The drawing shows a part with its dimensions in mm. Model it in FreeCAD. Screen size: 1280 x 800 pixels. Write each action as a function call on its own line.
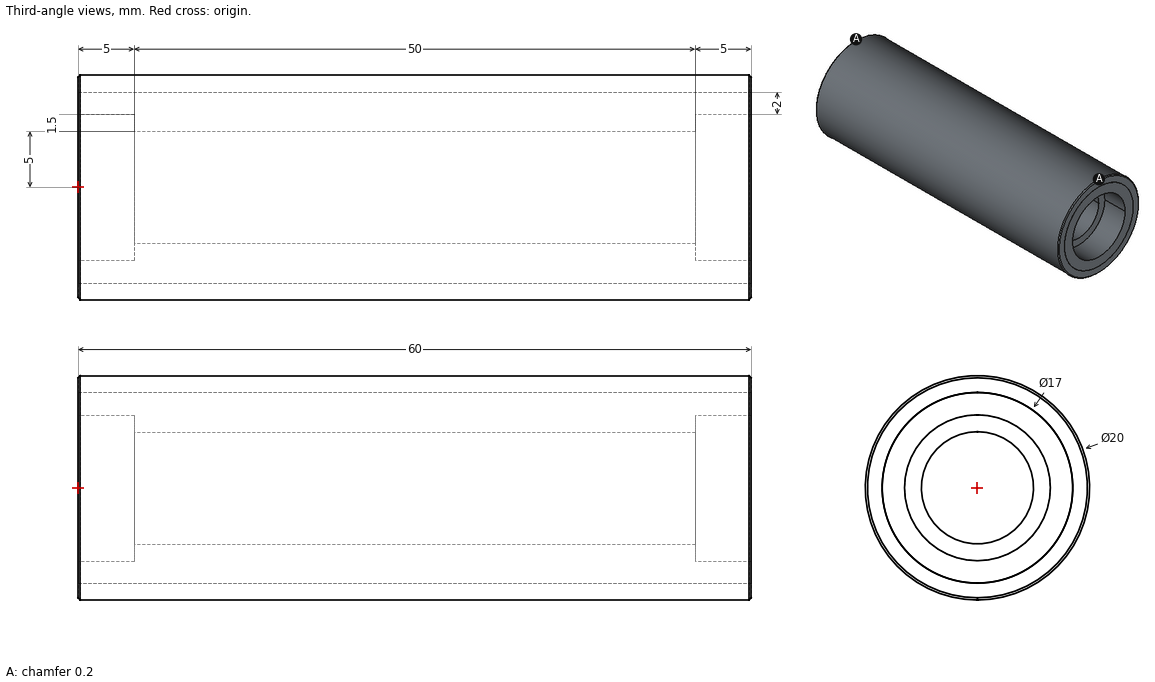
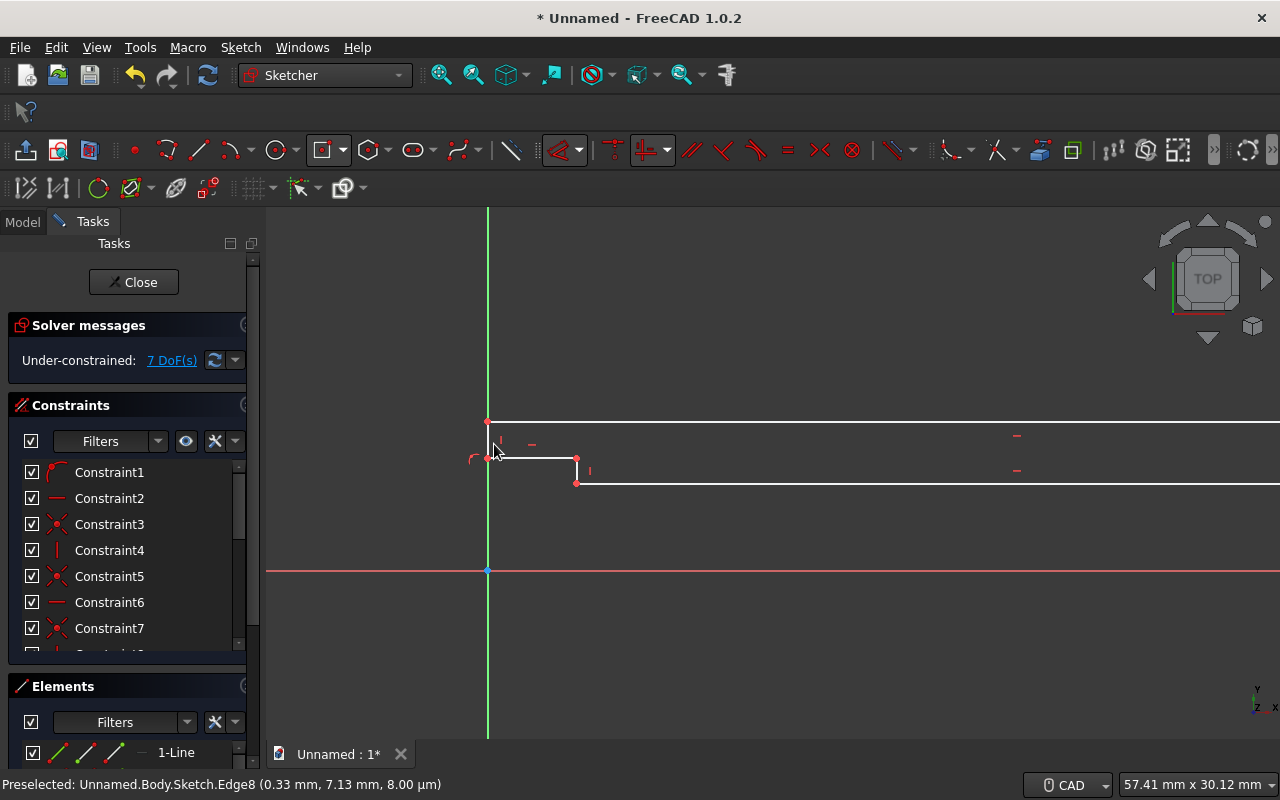
click(514, 458)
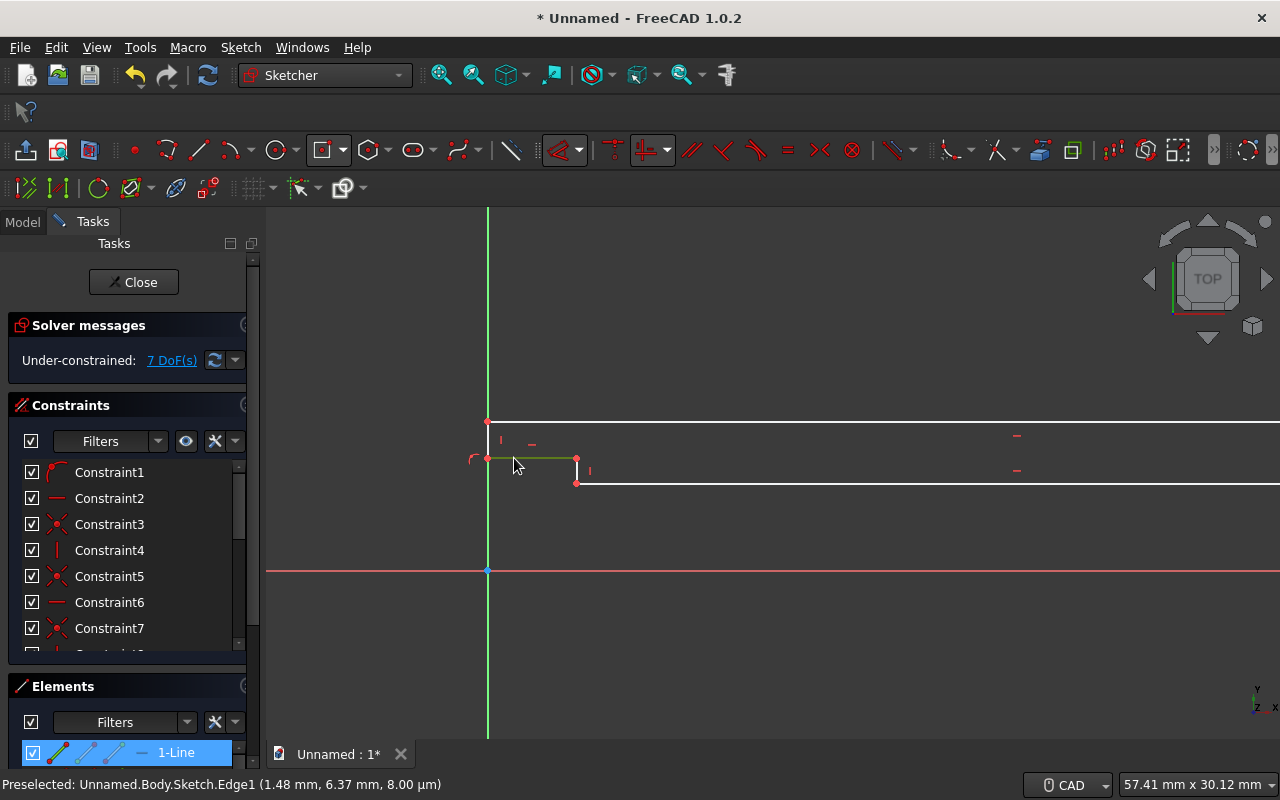
key(l)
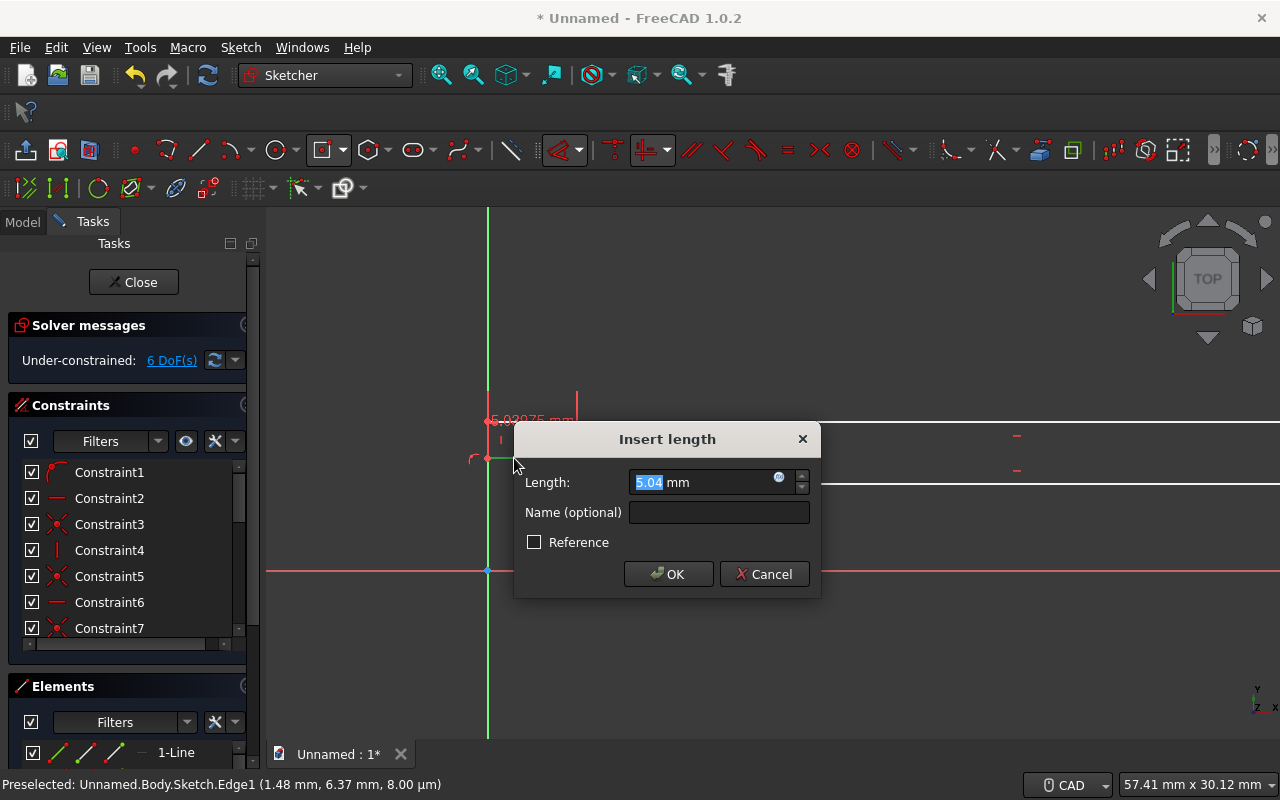
text(5)
key(Return)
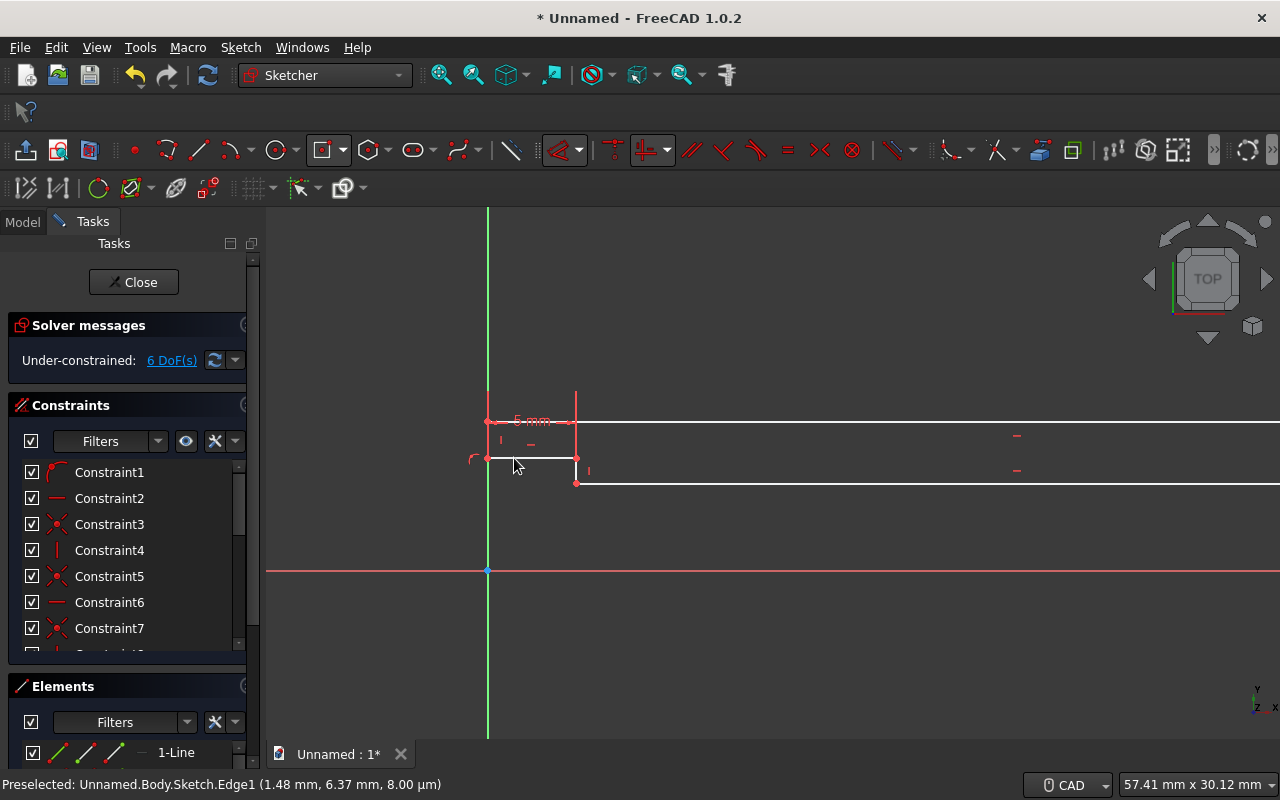
scroll(324, 445, down, 3)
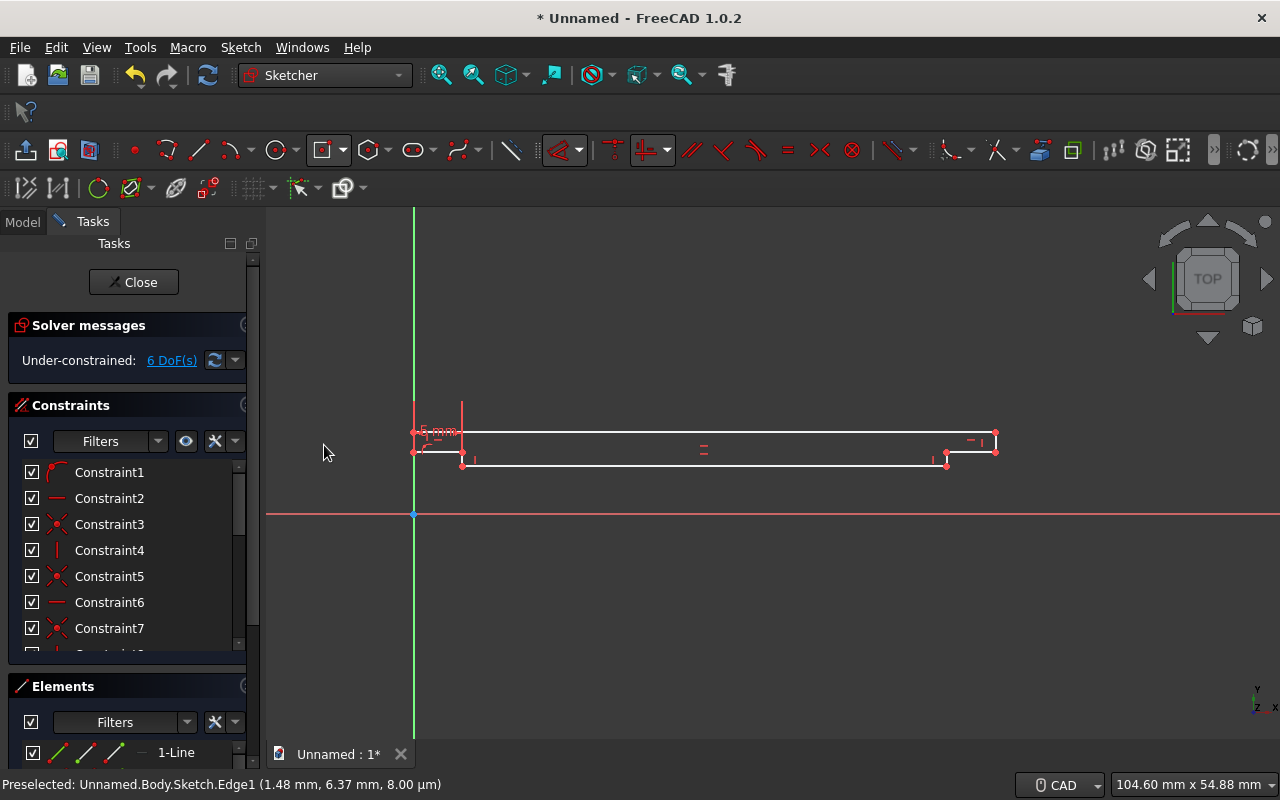
click(961, 452)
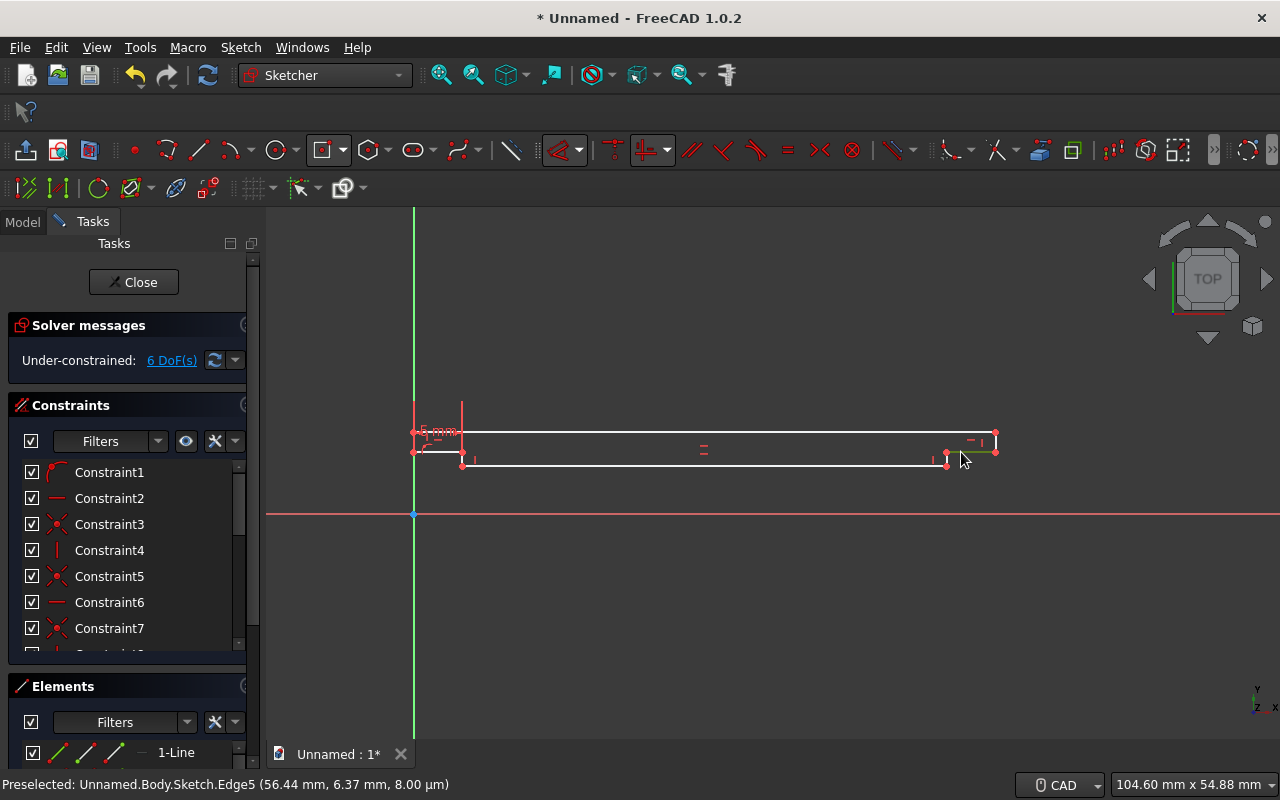
click(582, 150)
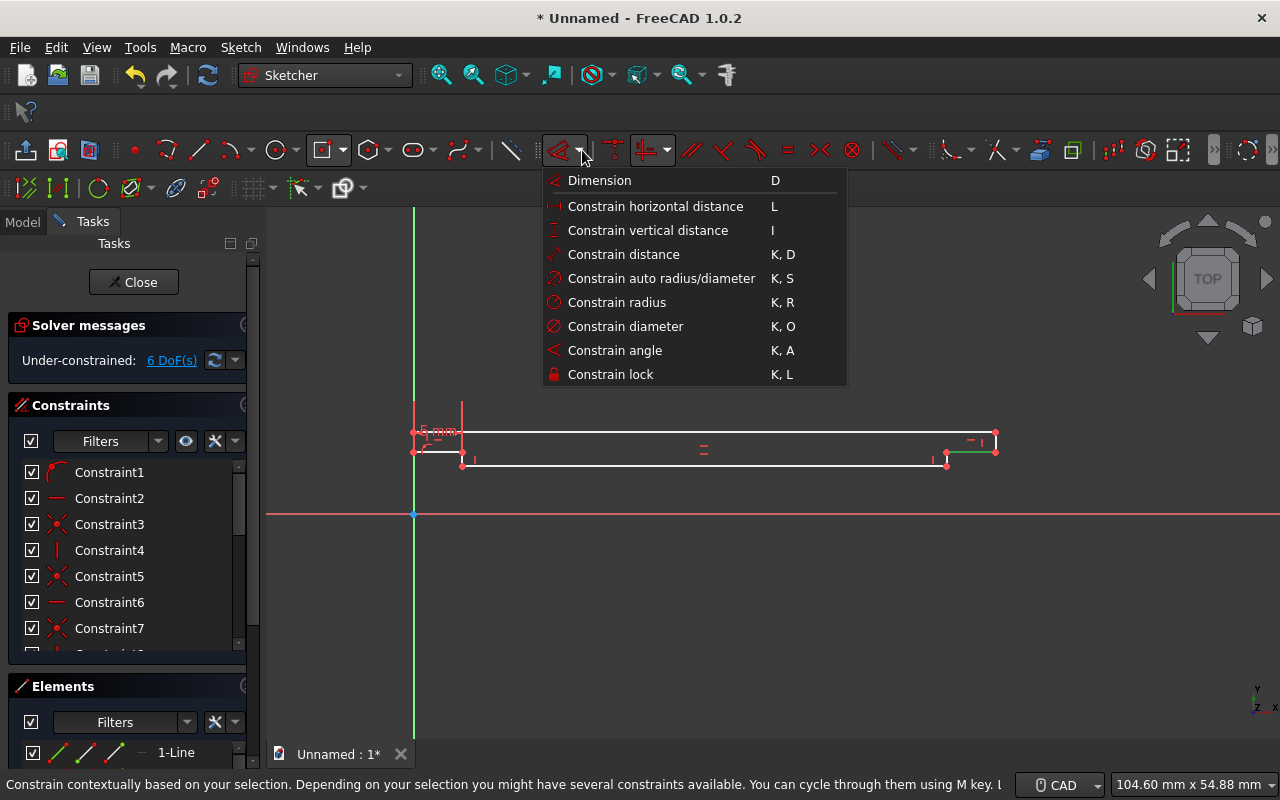
click(695, 206)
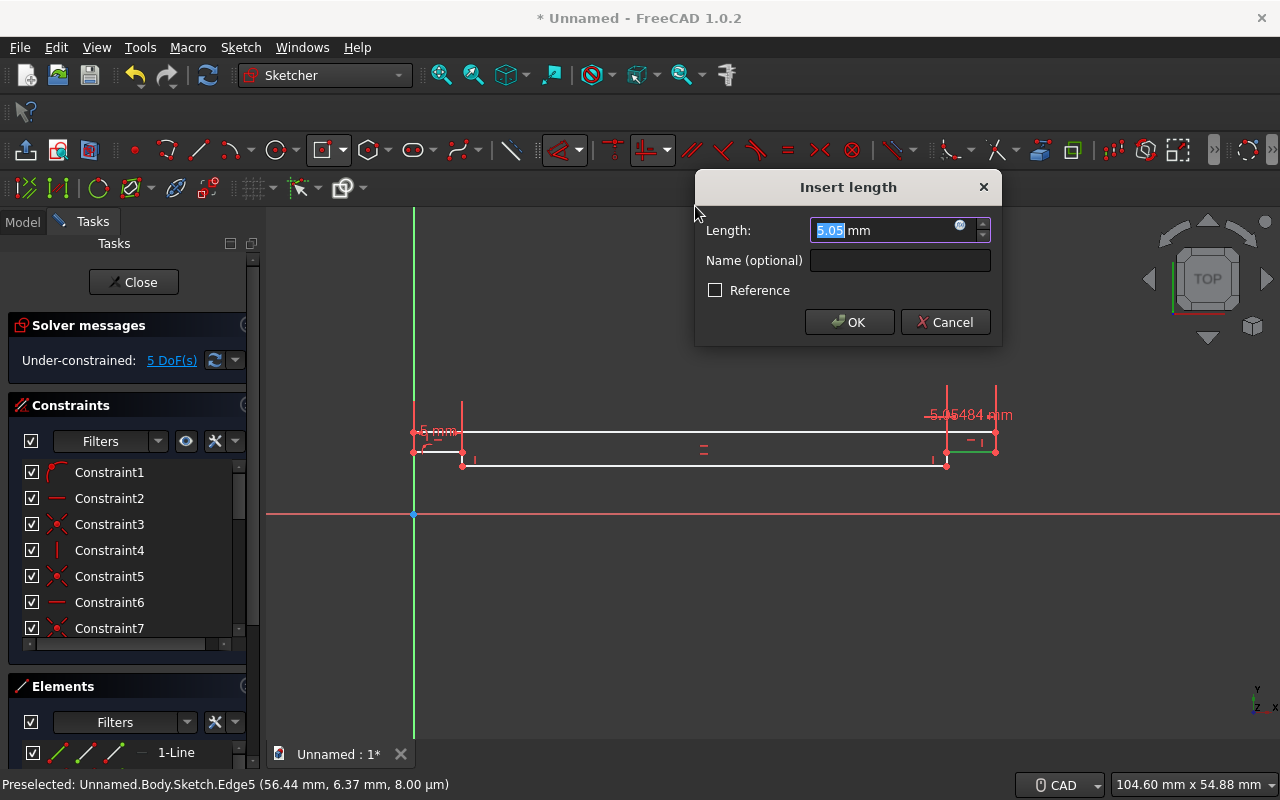
text(5)
key(Return)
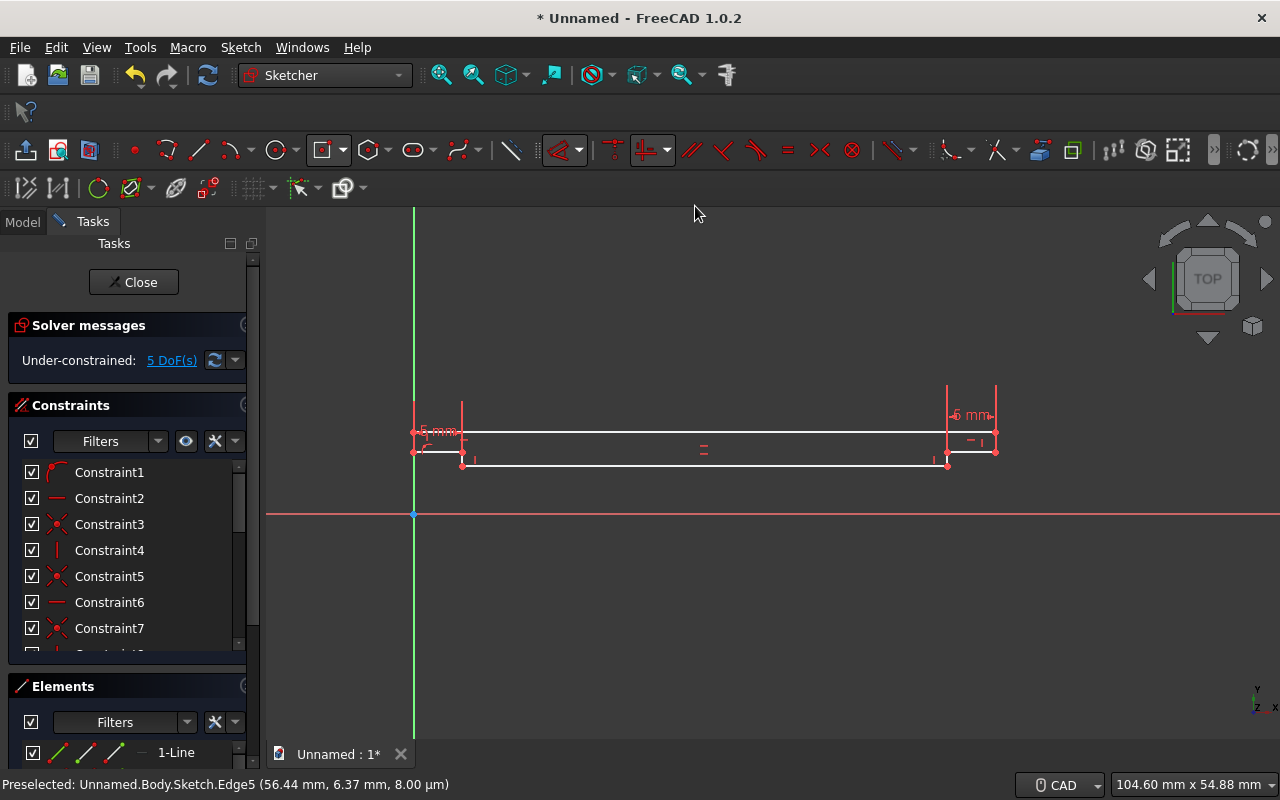
scroll(996, 442, up, 4)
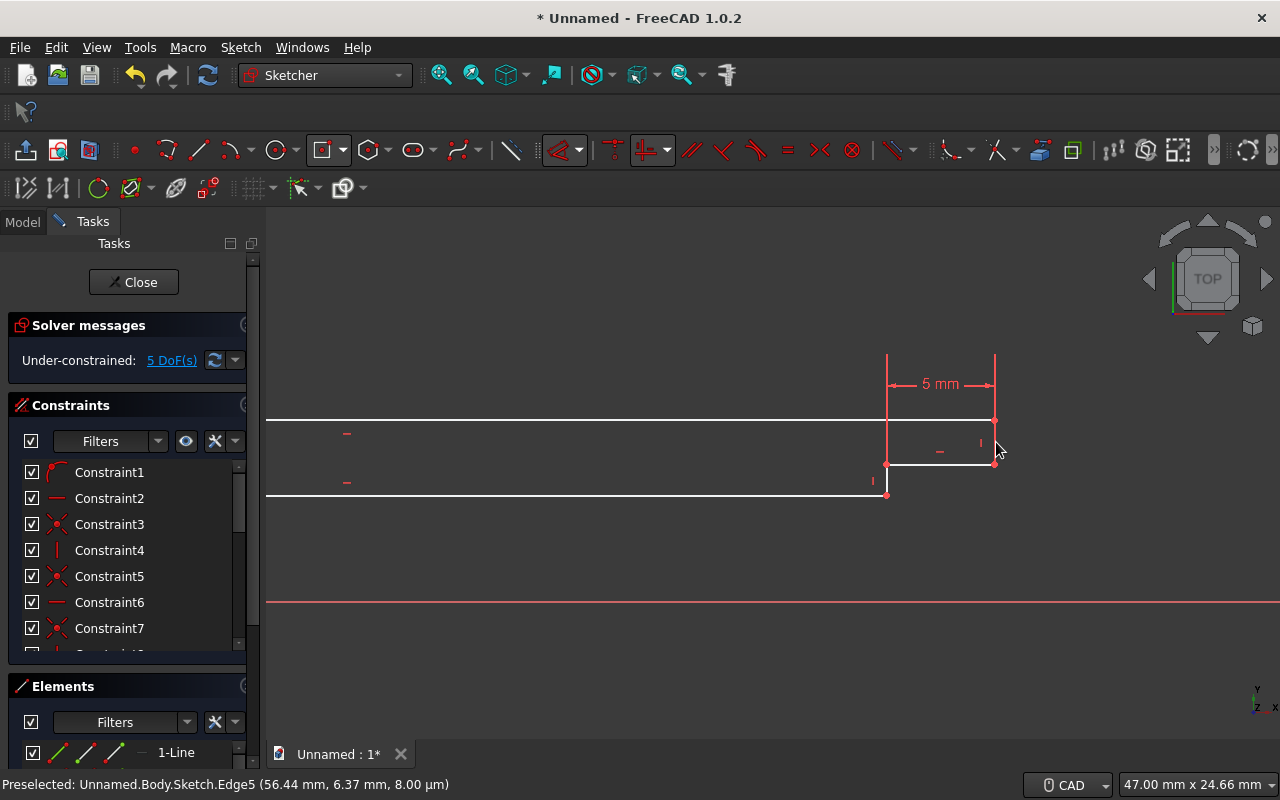
click(995, 442)